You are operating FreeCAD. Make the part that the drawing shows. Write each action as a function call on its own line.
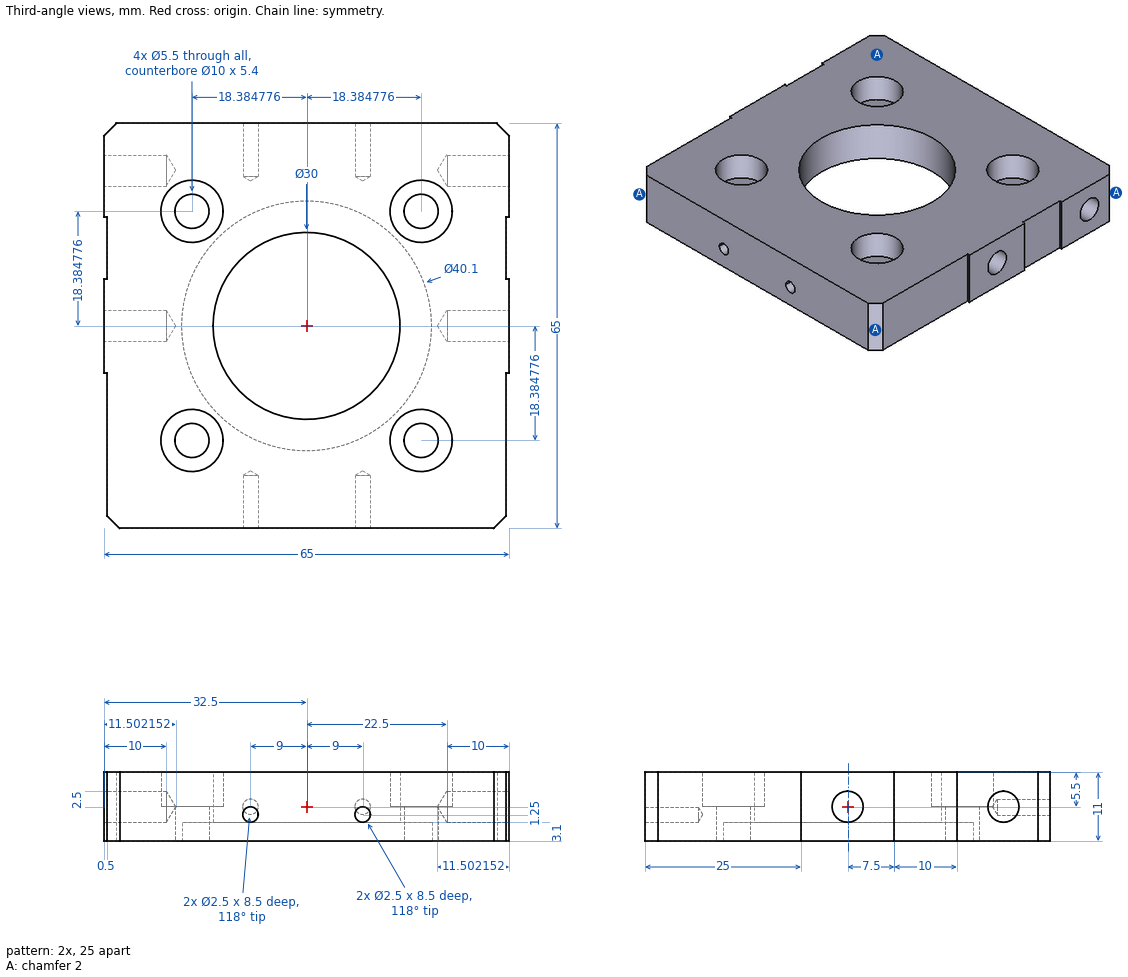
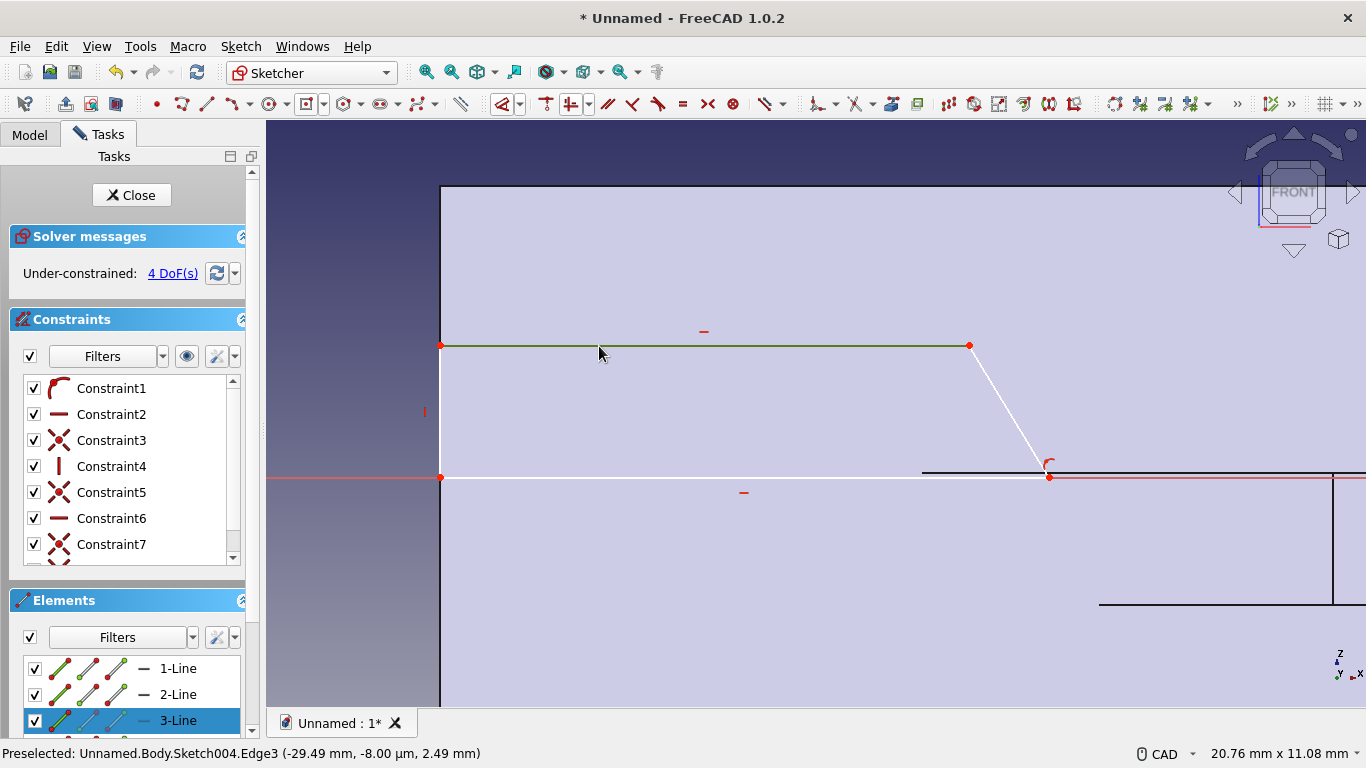
click(520, 104)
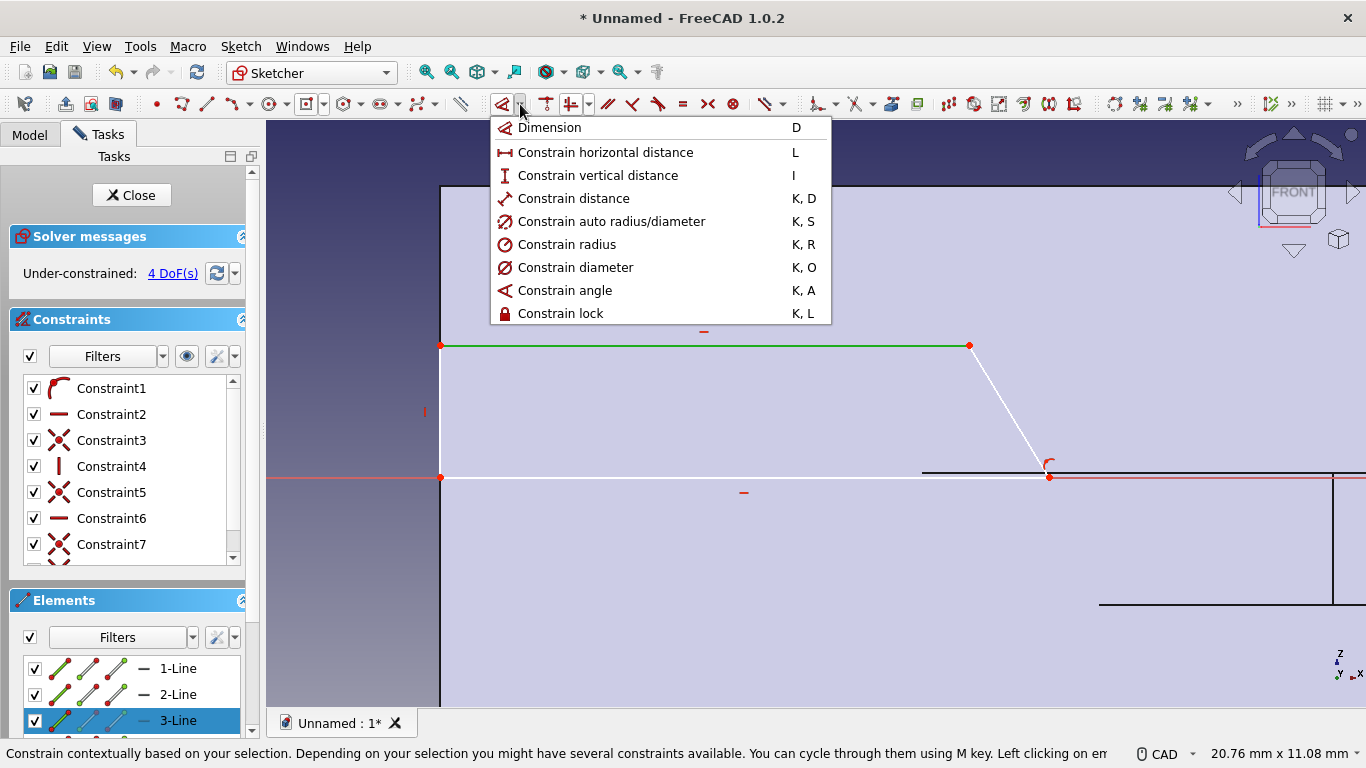
click(661, 152)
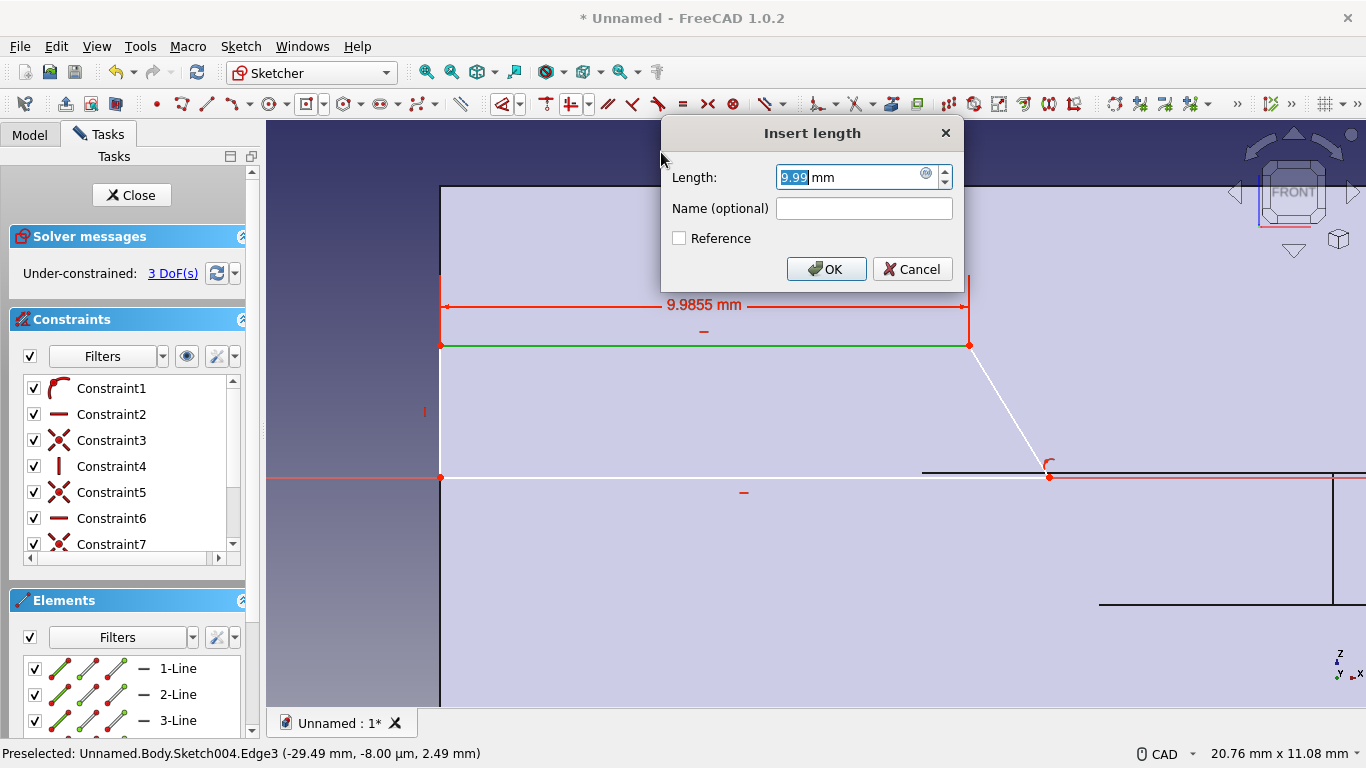
text(10)
key(Return)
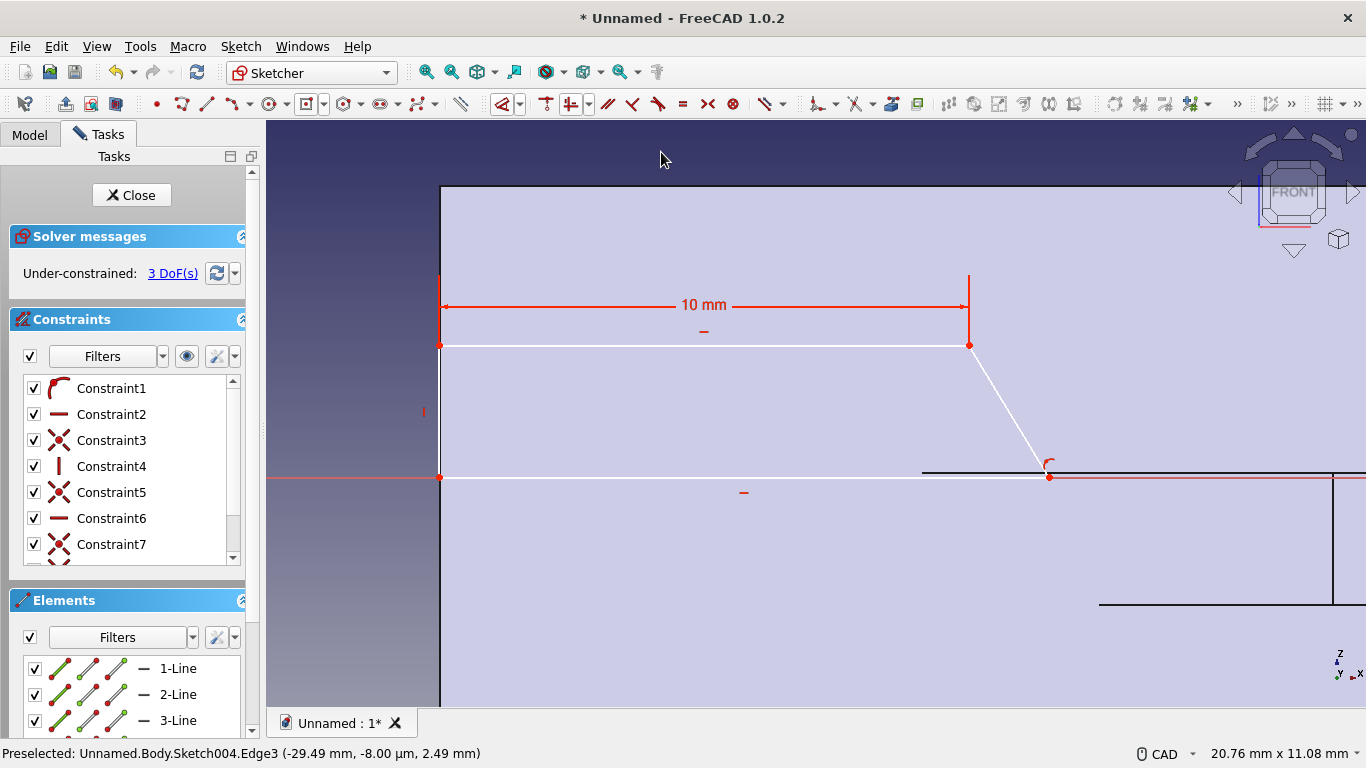
click(439, 438)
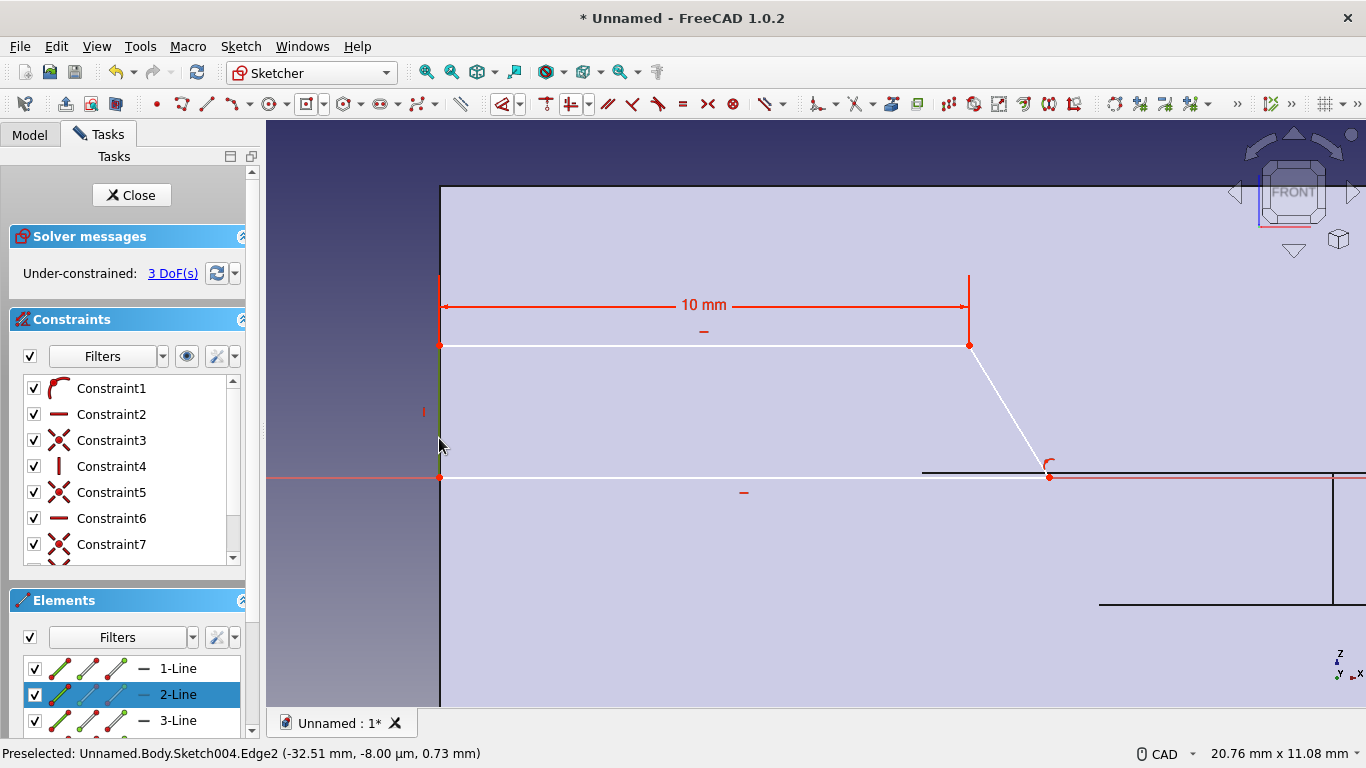
key(i)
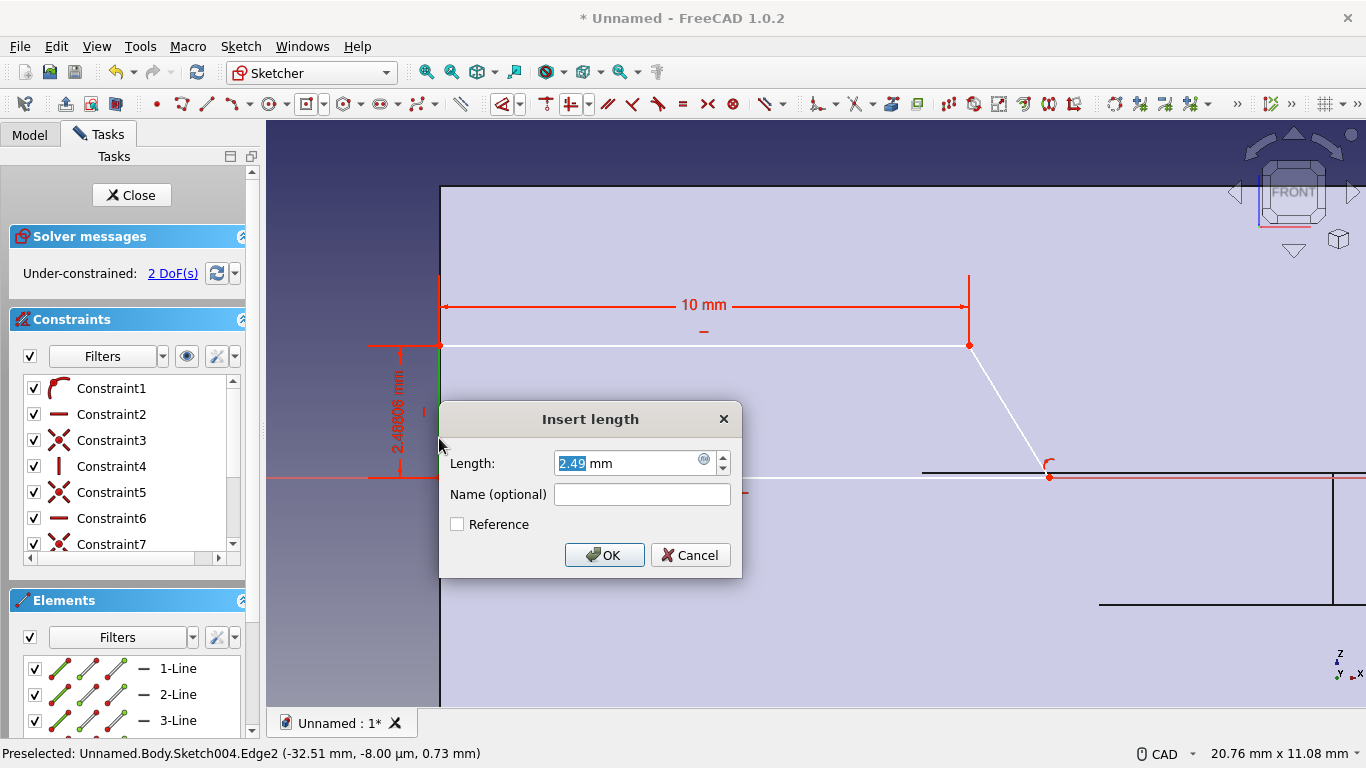
text(2.5)
key(Return)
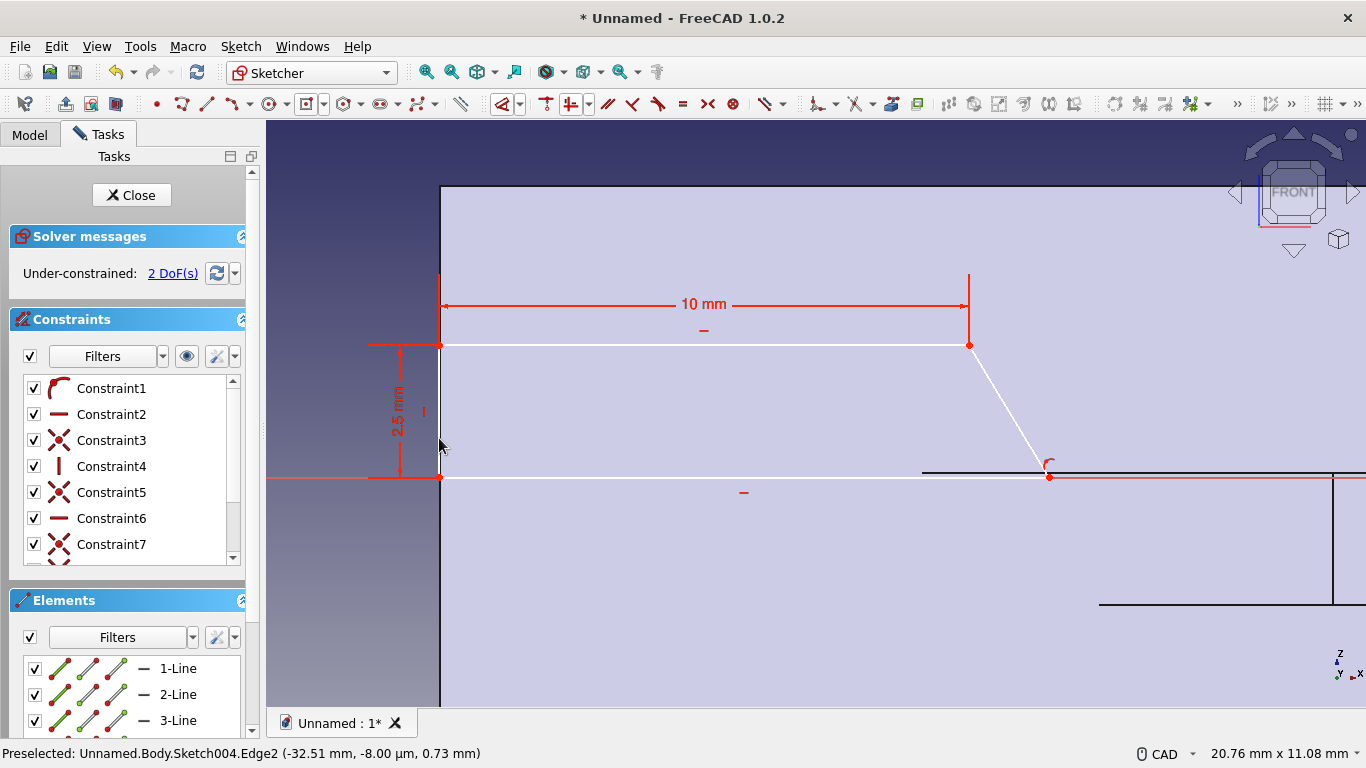
click(439, 478)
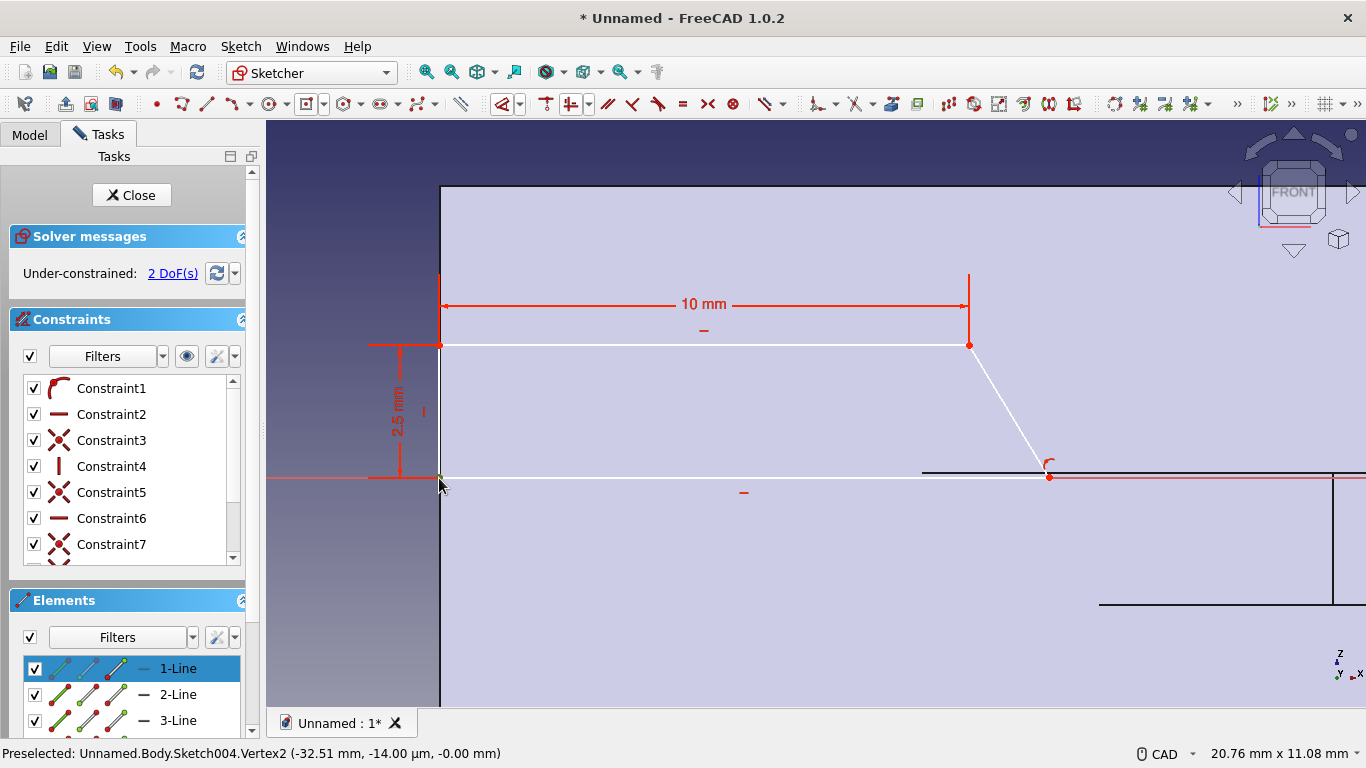
click(520, 104)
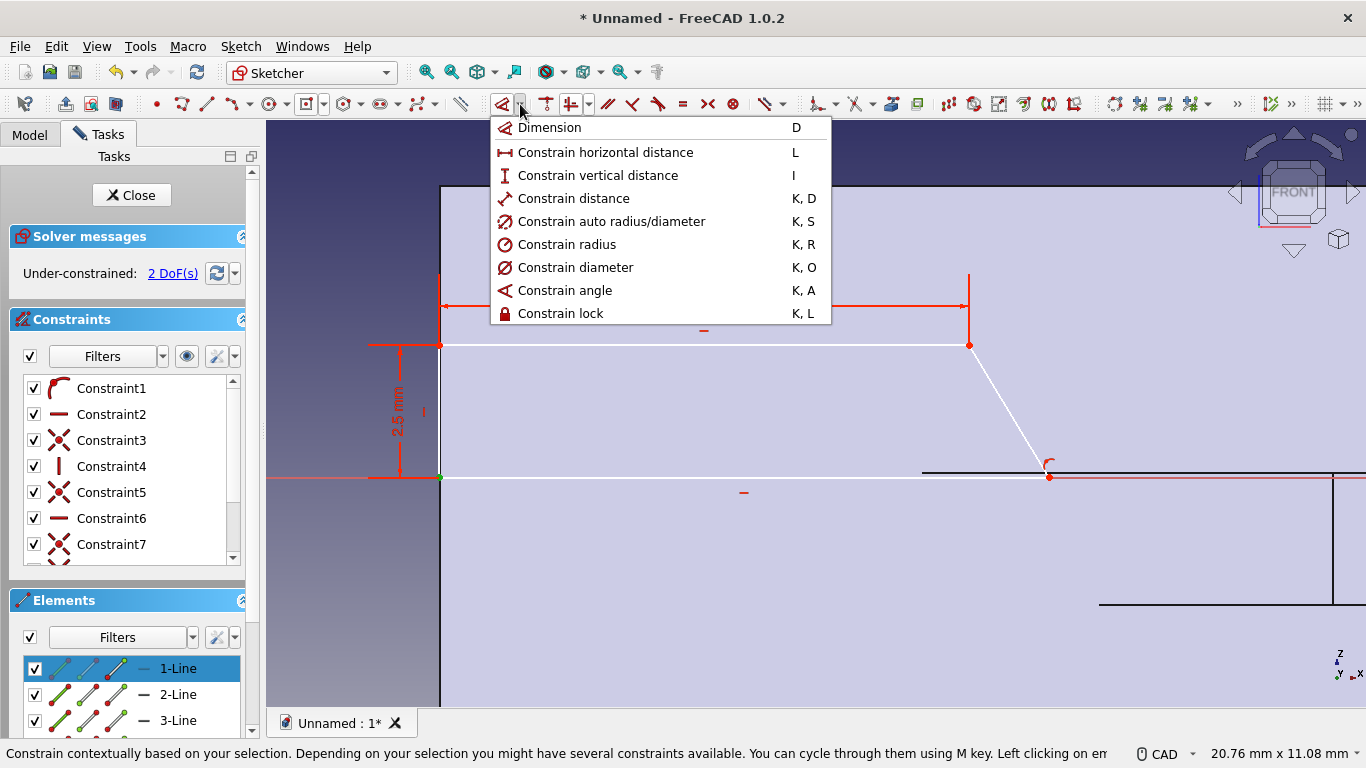
click(661, 152)